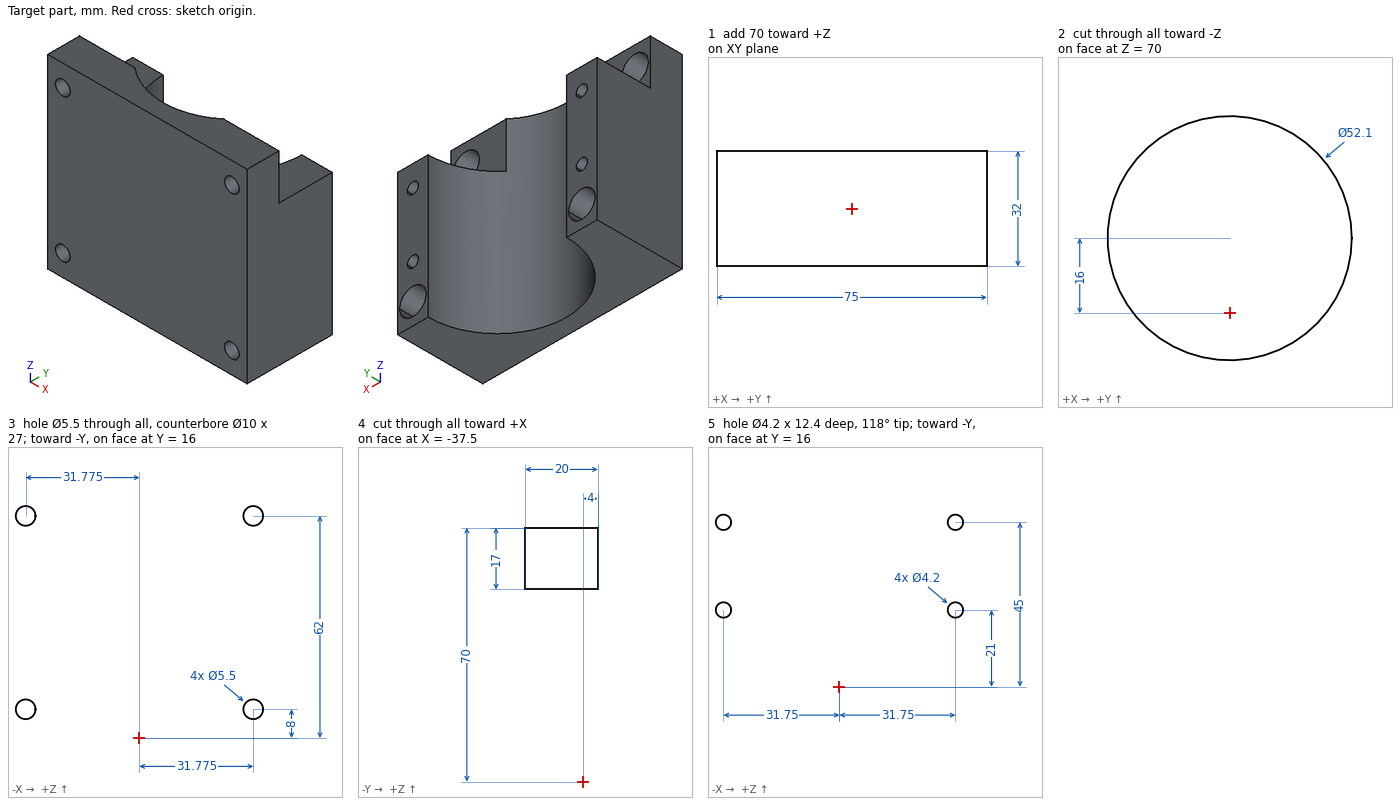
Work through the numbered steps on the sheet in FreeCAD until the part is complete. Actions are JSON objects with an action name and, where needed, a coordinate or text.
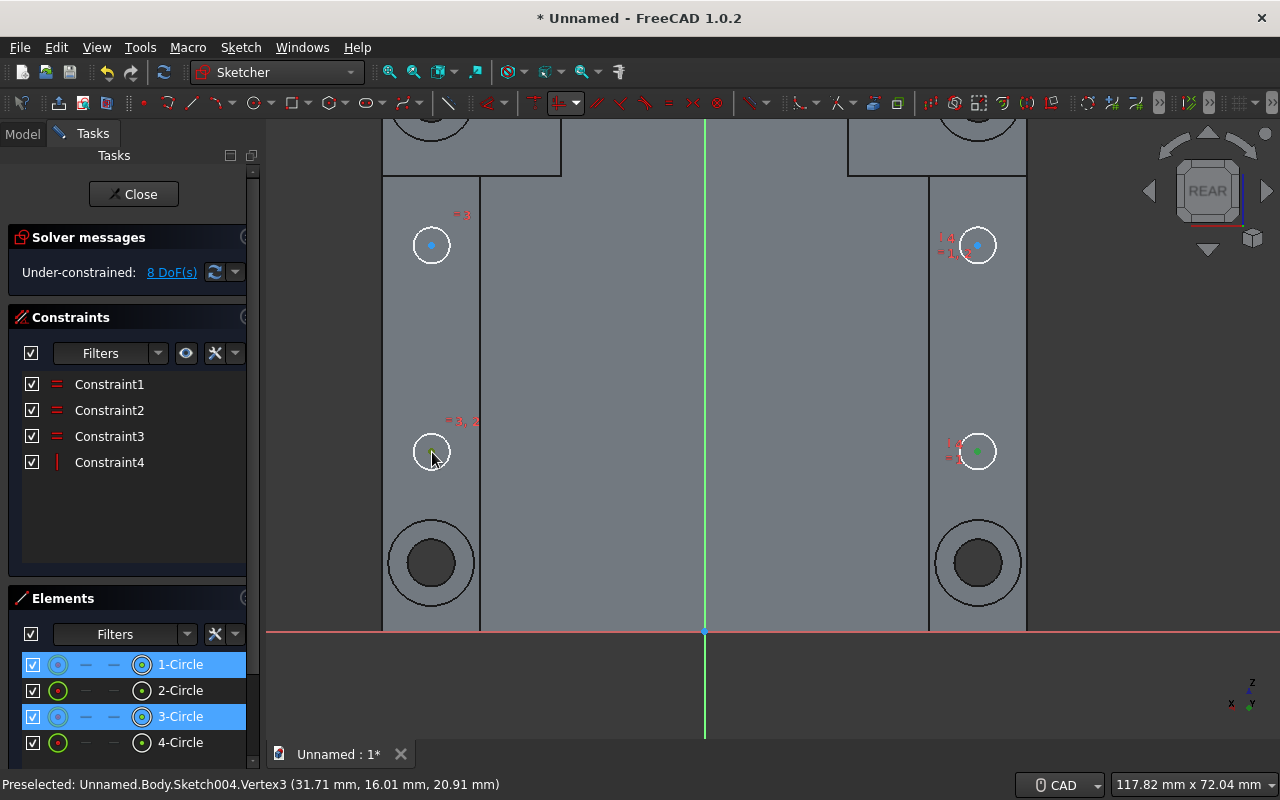
{"action": "left_click", "coordinate": [578, 104]}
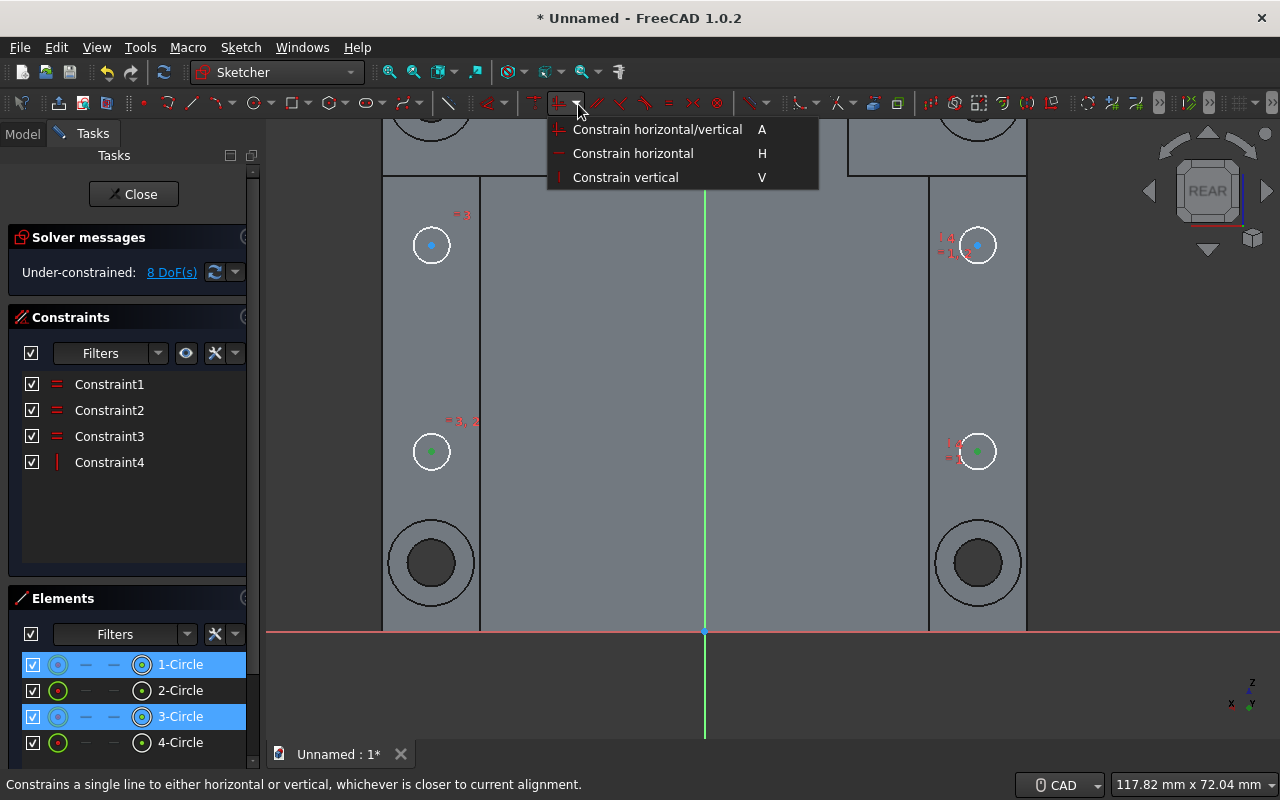
{"action": "left_click", "coordinate": [683, 153]}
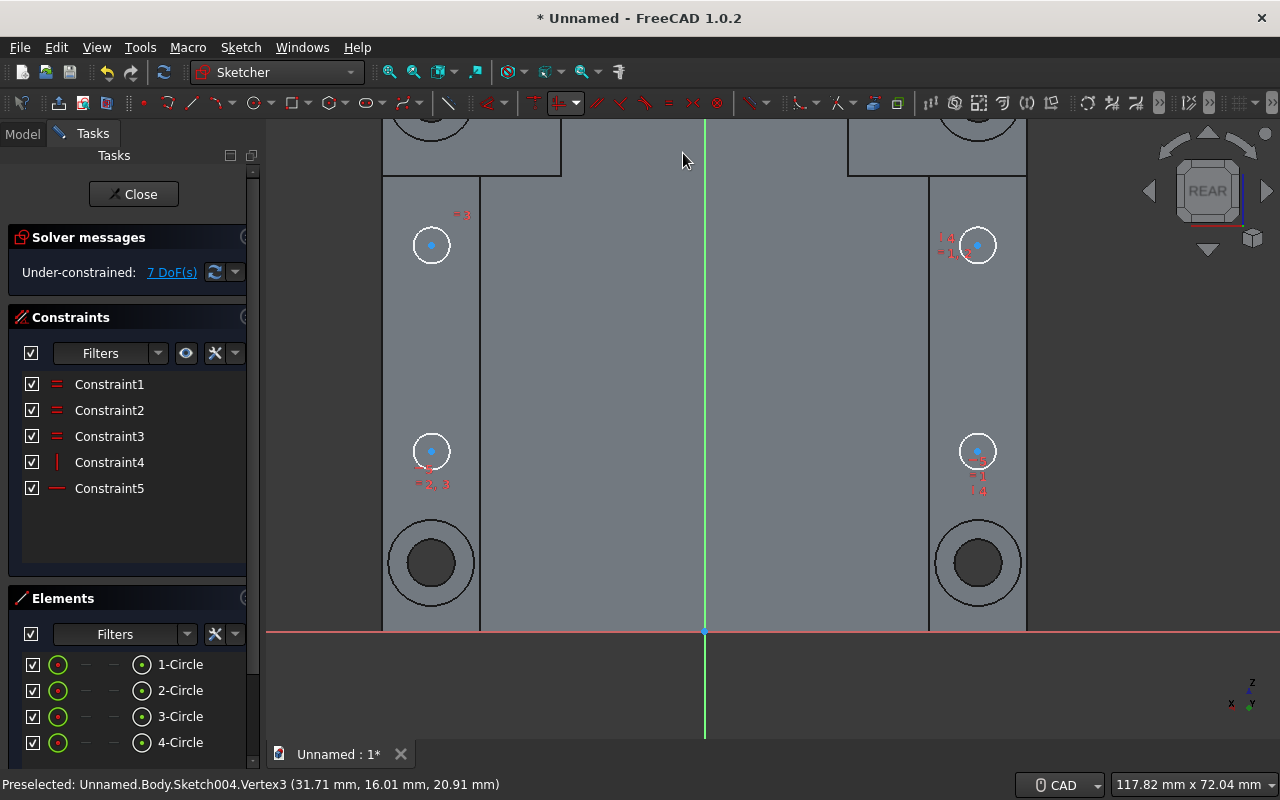
{"action": "left_click", "coordinate": [432, 452]}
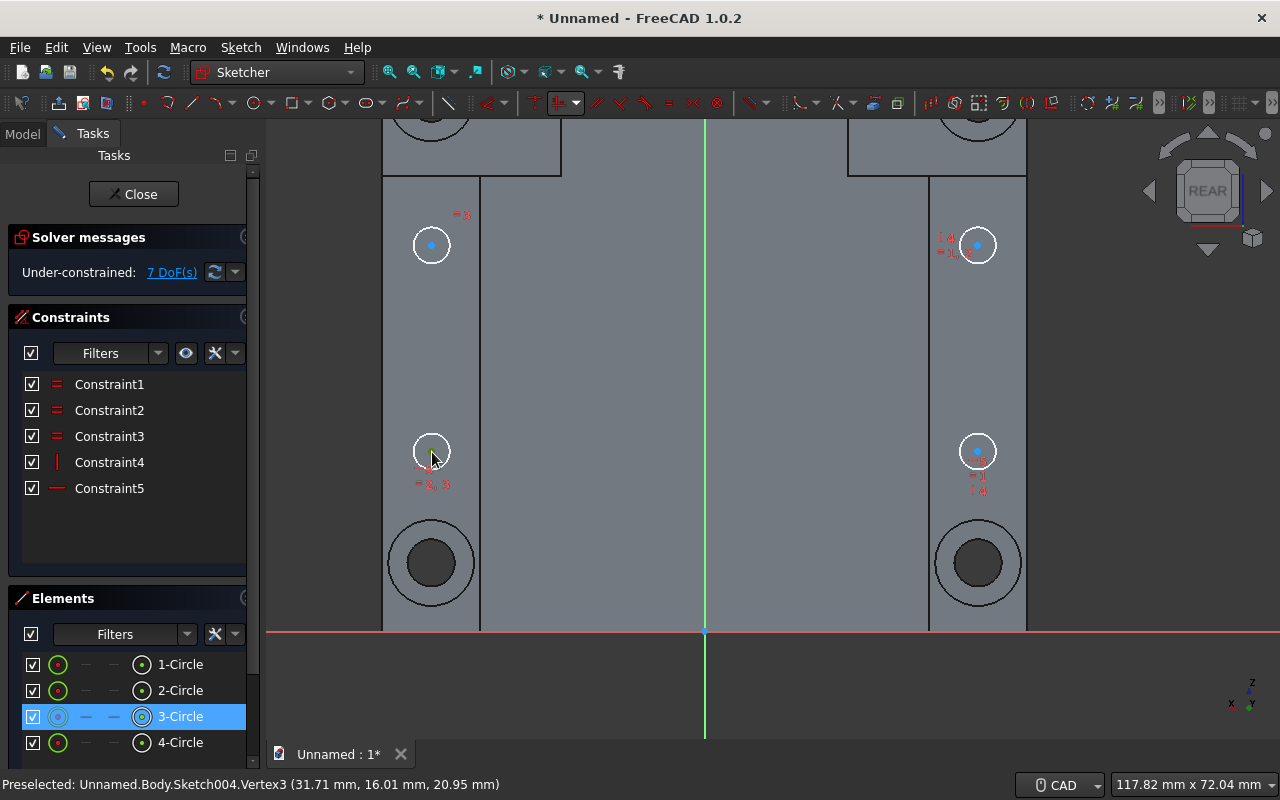
{"action": "left_click", "coordinate": [432, 245]}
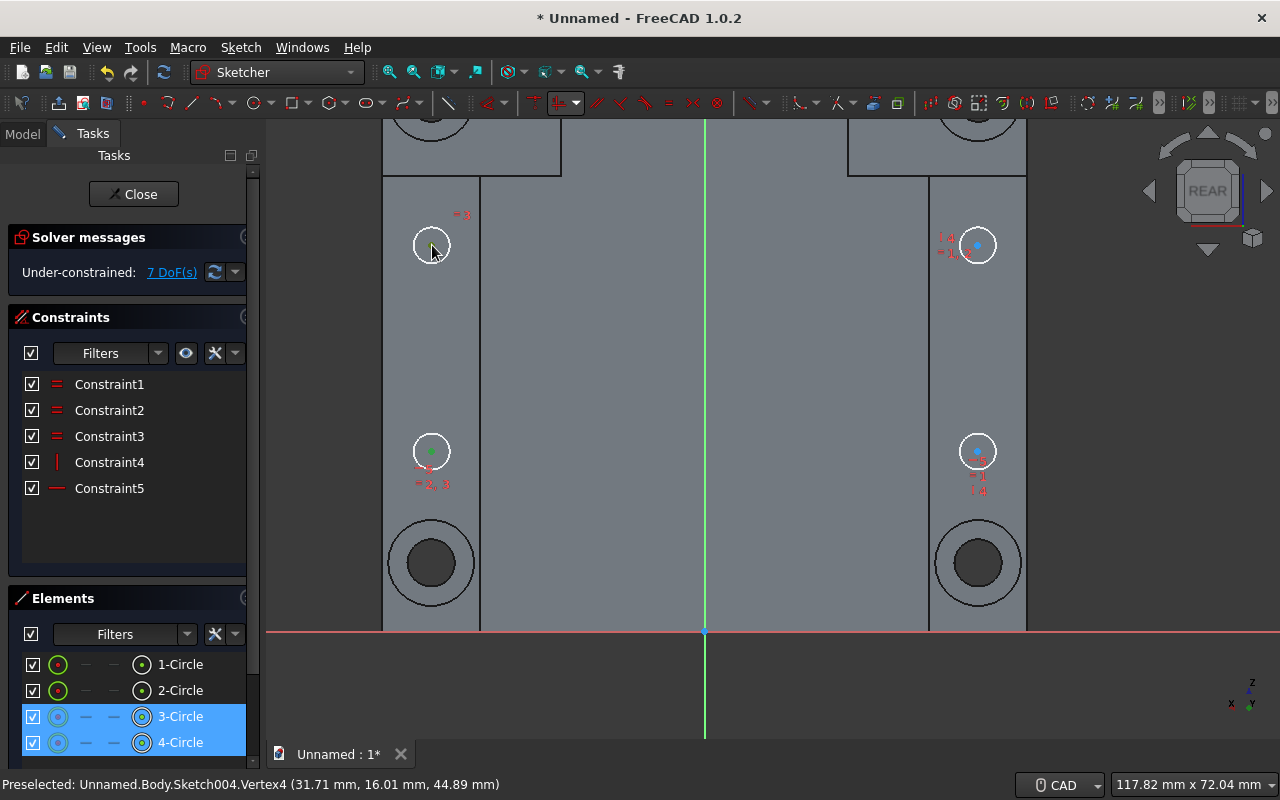
{"action": "key", "text": "v"}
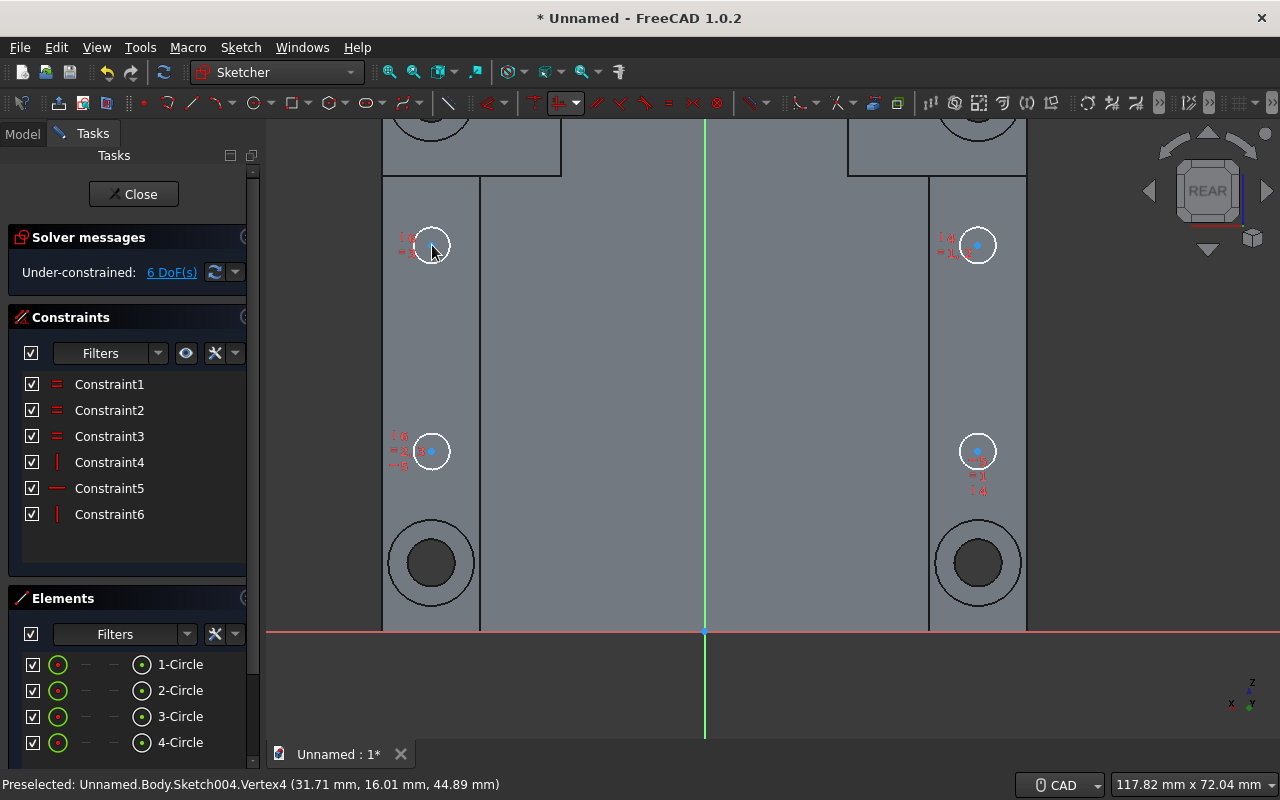
{"action": "left_click", "coordinate": [978, 245]}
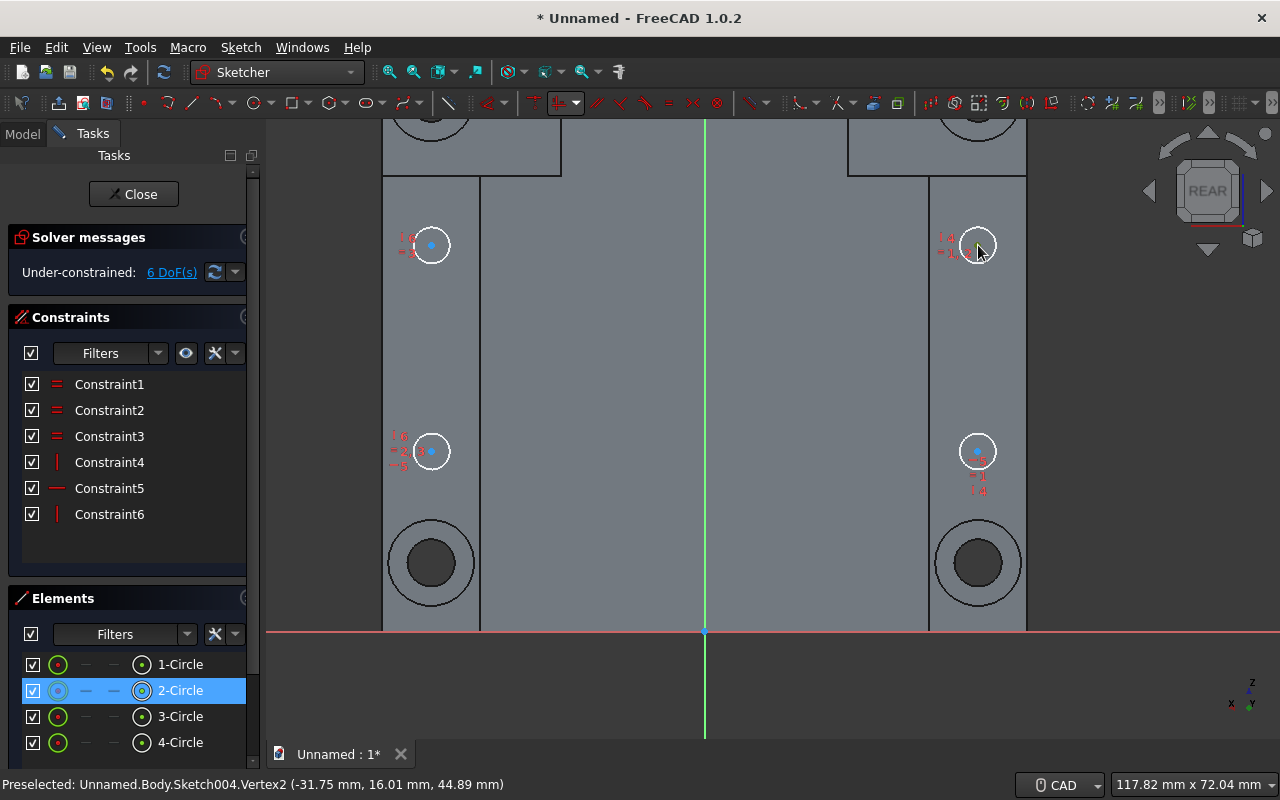
{"action": "left_click", "coordinate": [432, 245]}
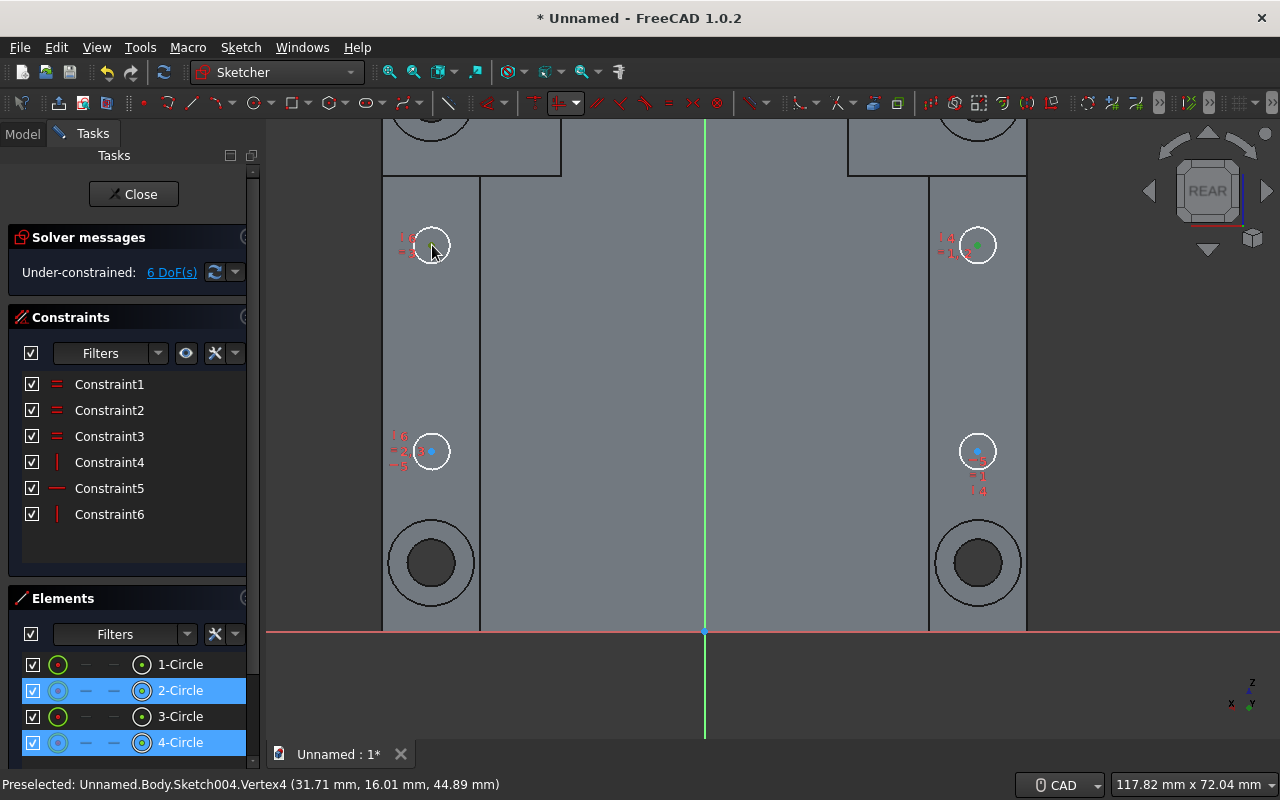
{"action": "key", "text": "h"}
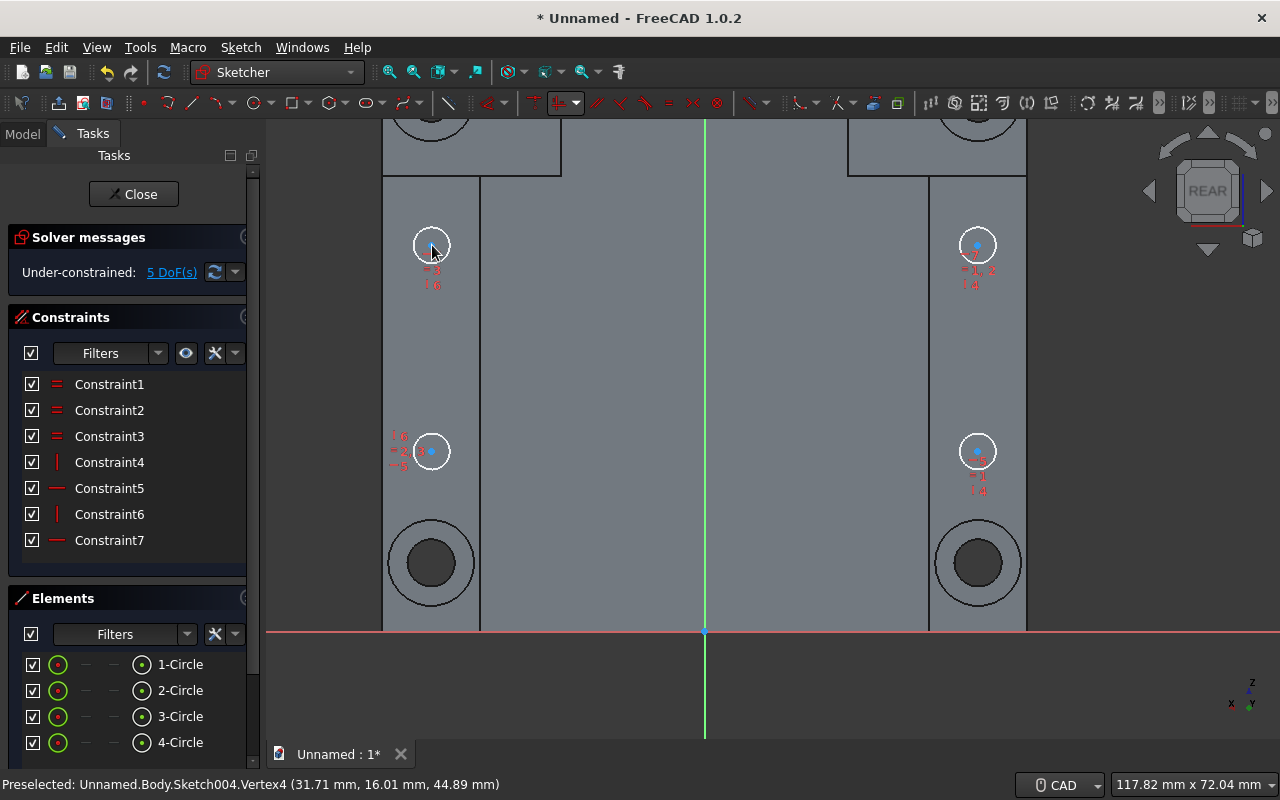
{"action": "left_click", "coordinate": [488, 104]}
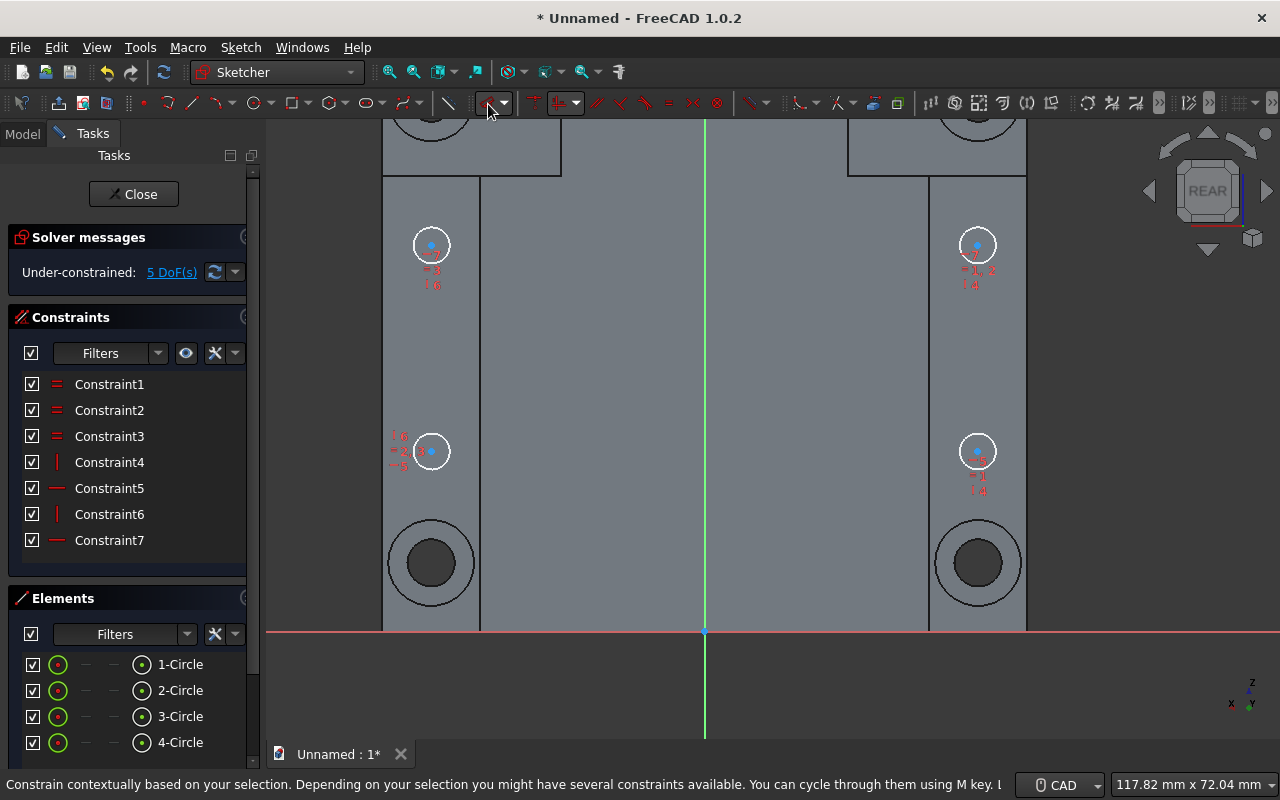
{"action": "left_click", "coordinate": [991, 439]}
{"action": "left_click", "coordinate": [1014, 417]}